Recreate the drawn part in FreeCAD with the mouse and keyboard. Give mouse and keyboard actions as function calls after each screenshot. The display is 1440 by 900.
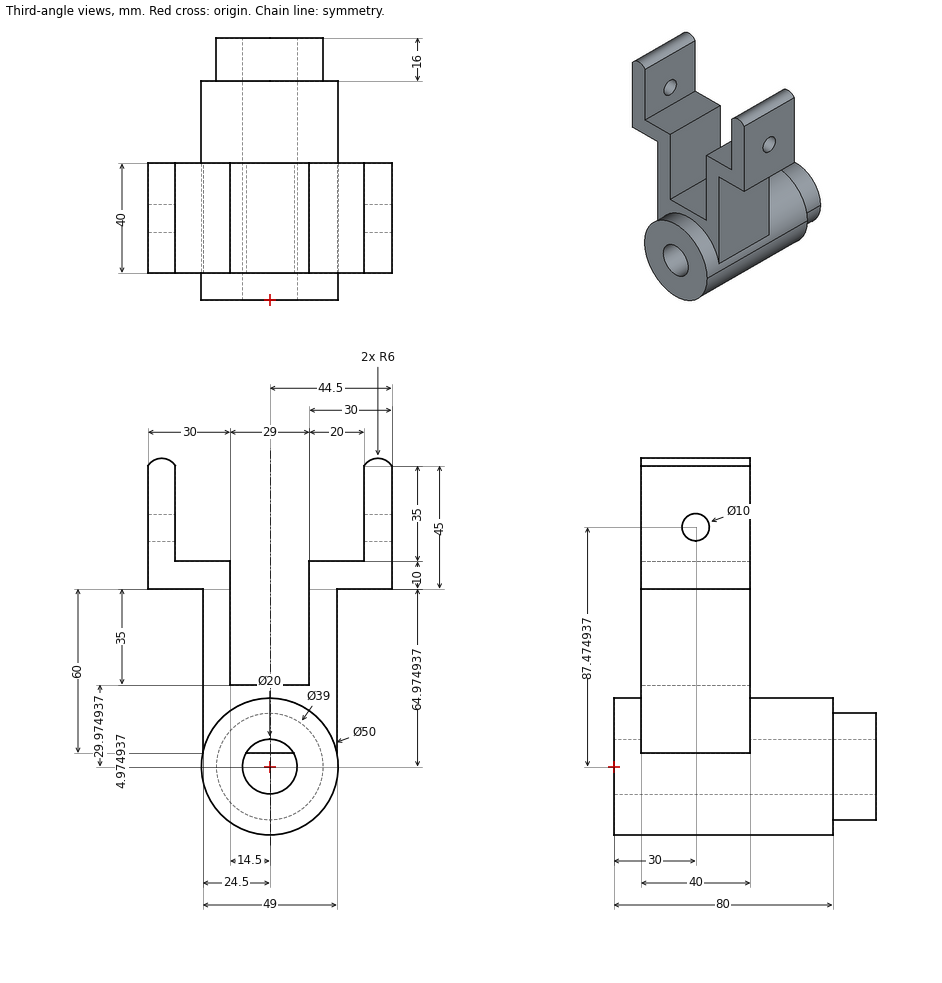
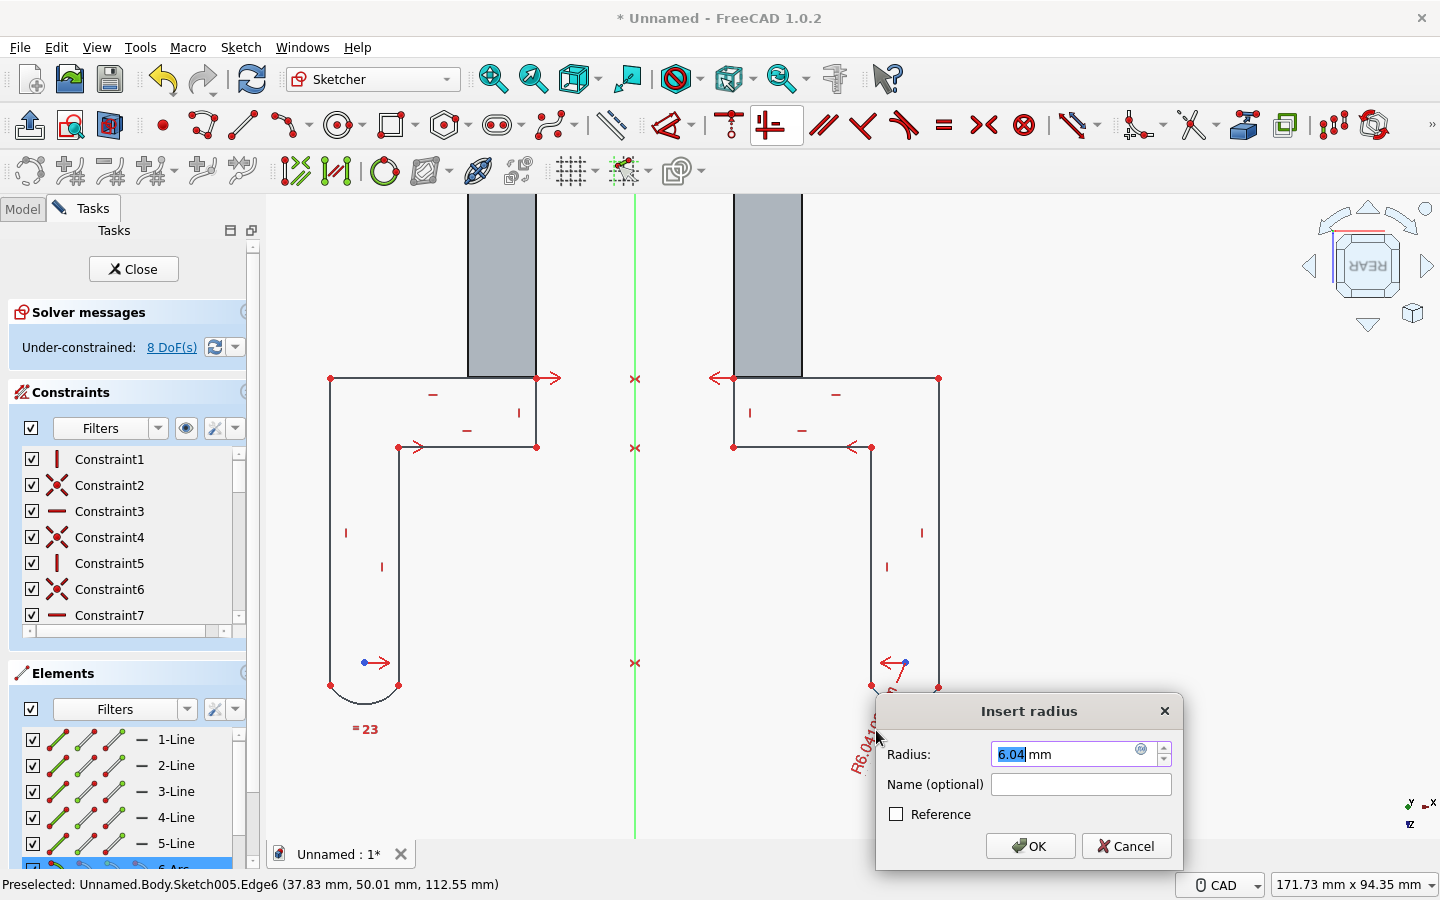
text(6)
key(Return)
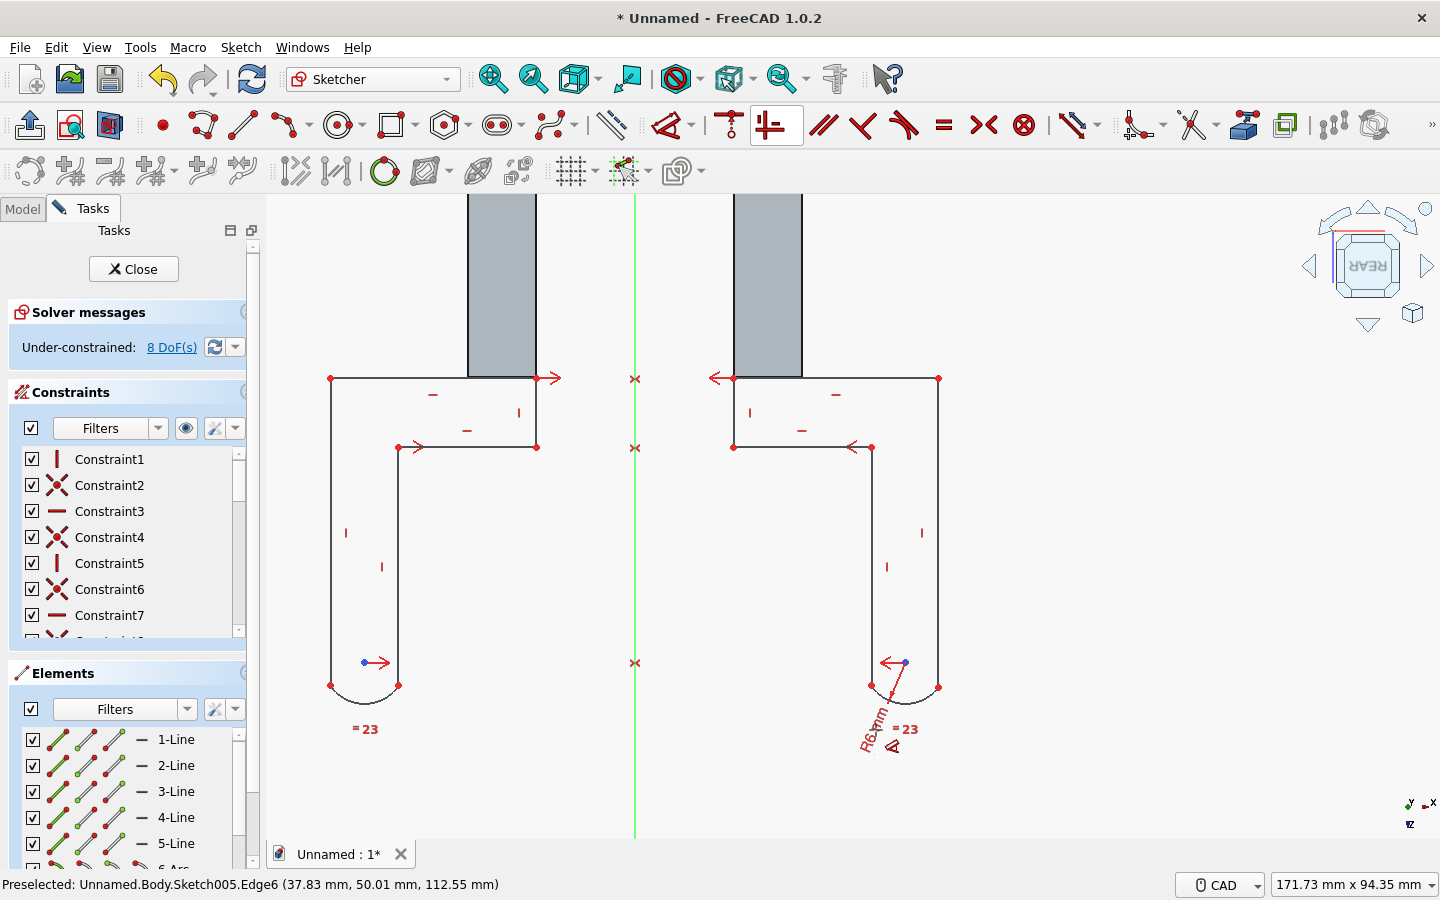
click(938, 595)
click(972, 533)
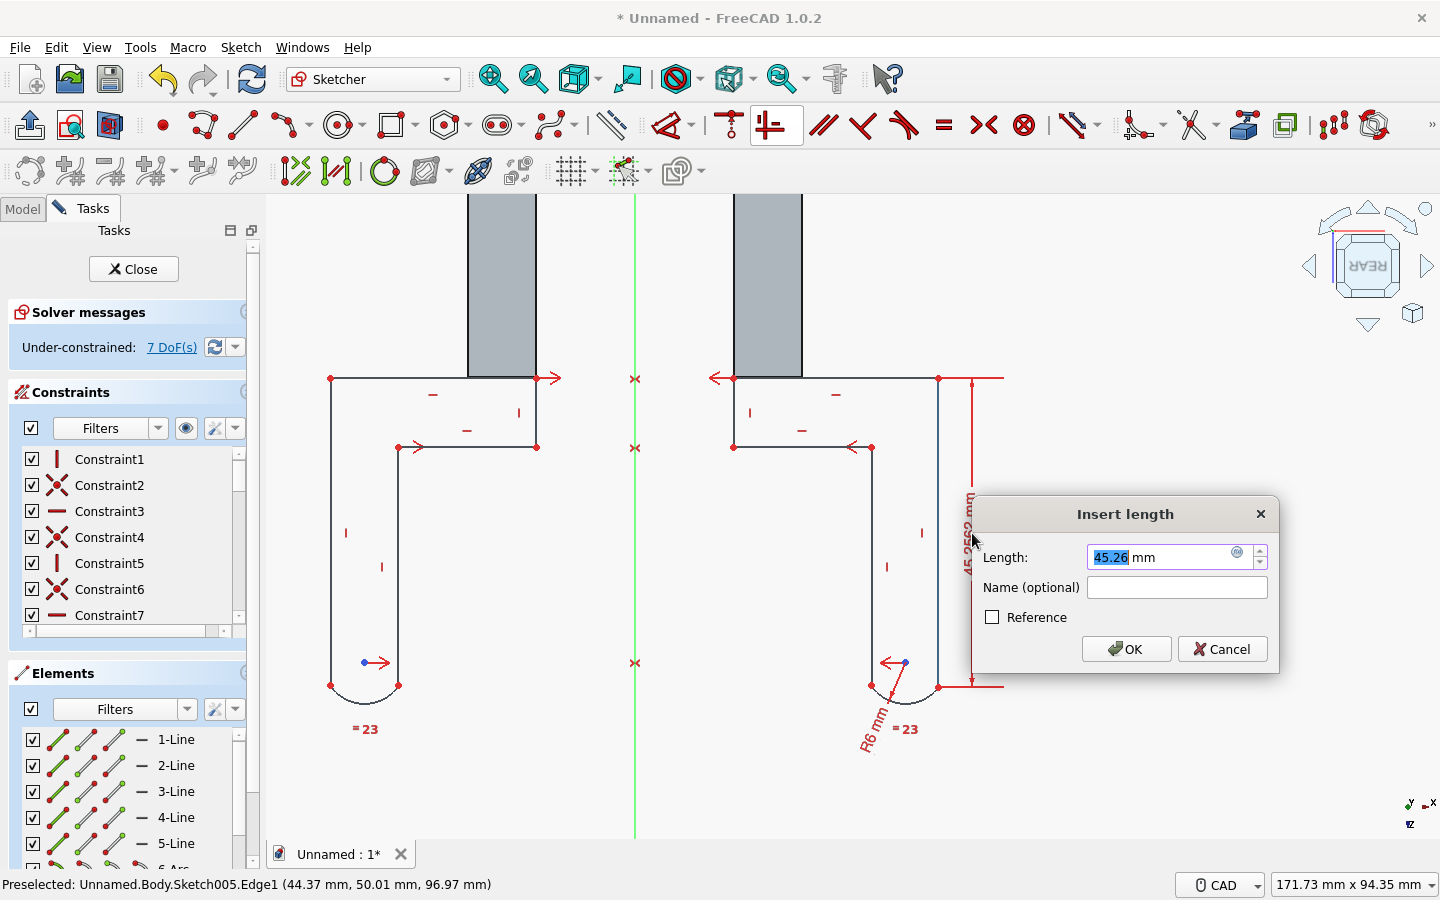
text(45)
key(Return)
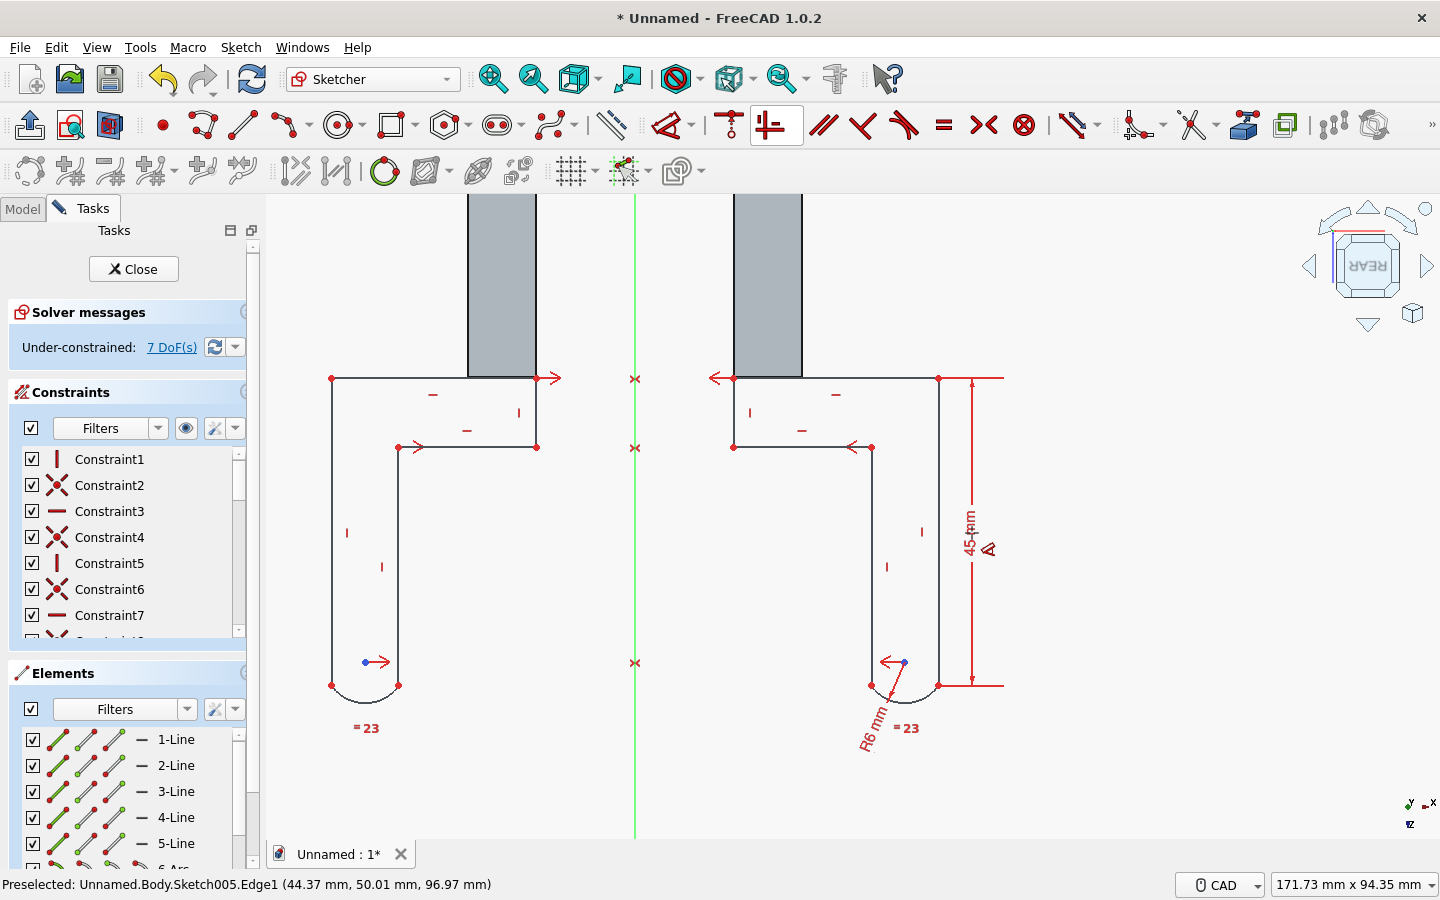
click(877, 378)
click(836, 412)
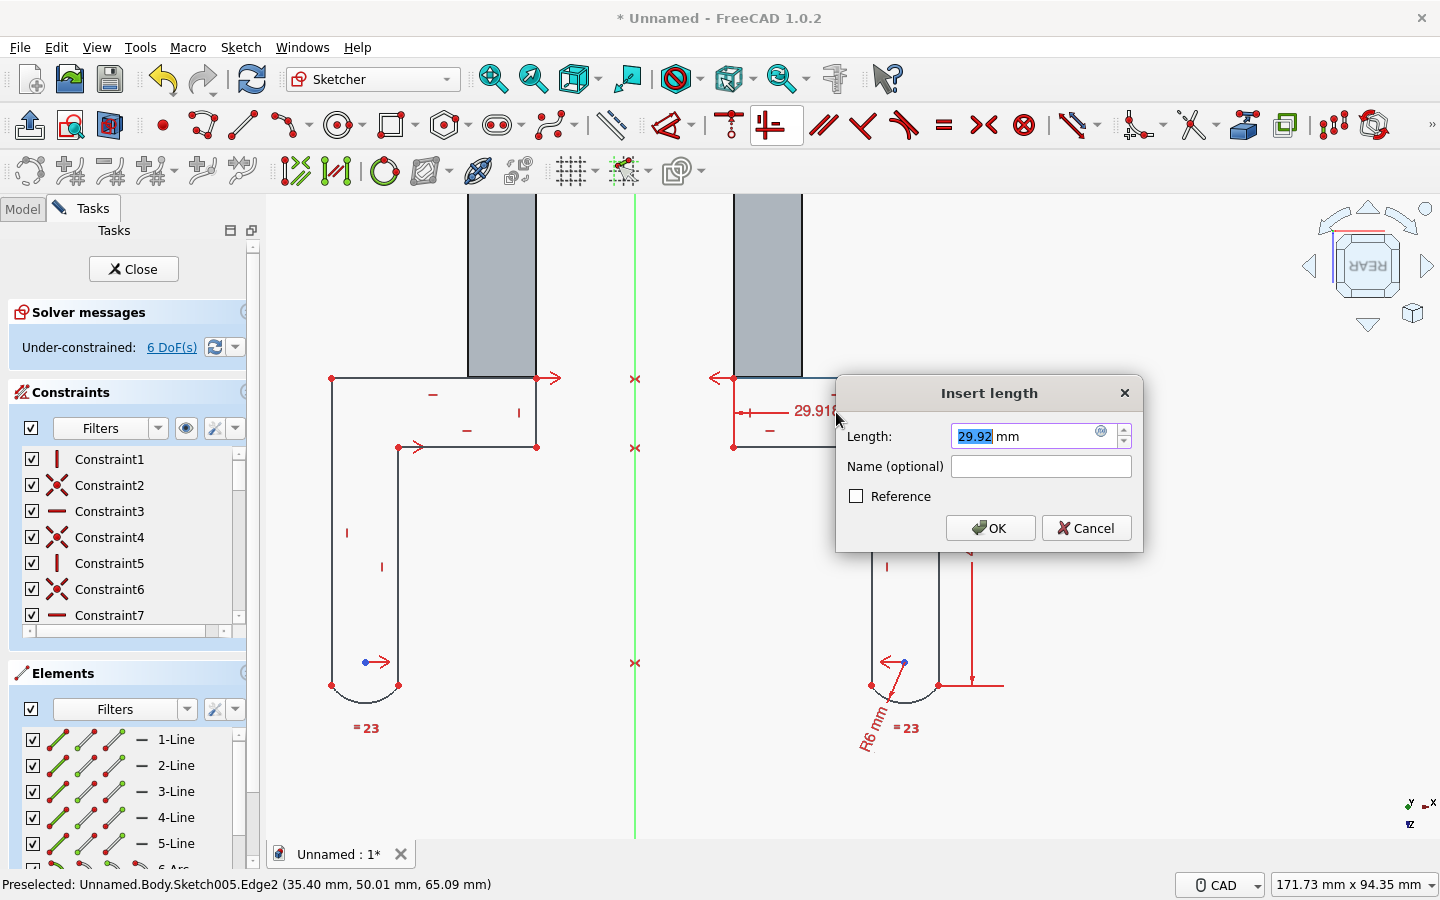
text(30)
key(Return)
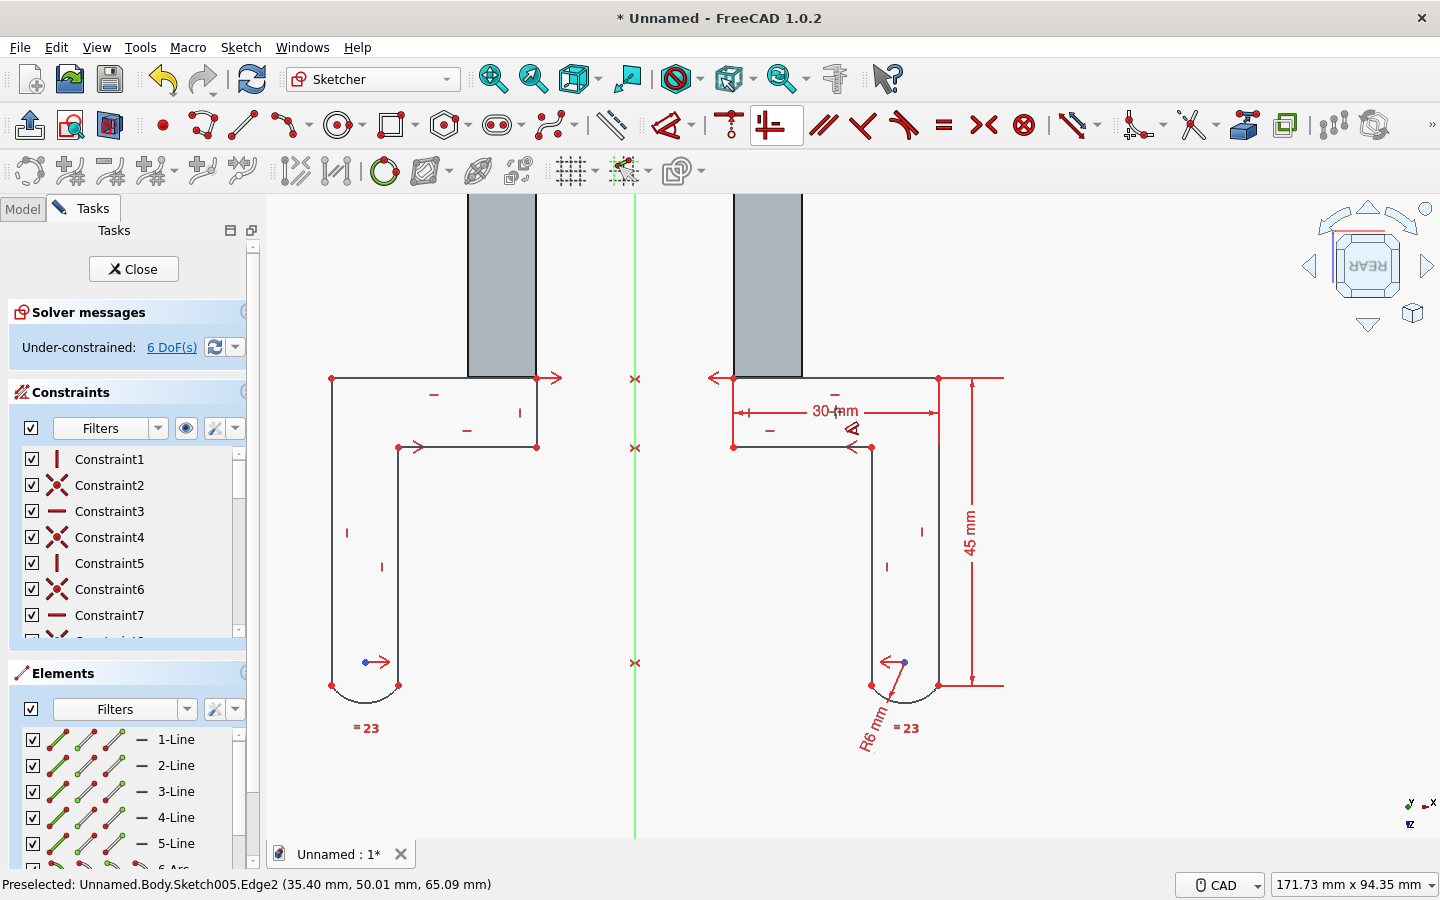
click(733, 399)
click(699, 413)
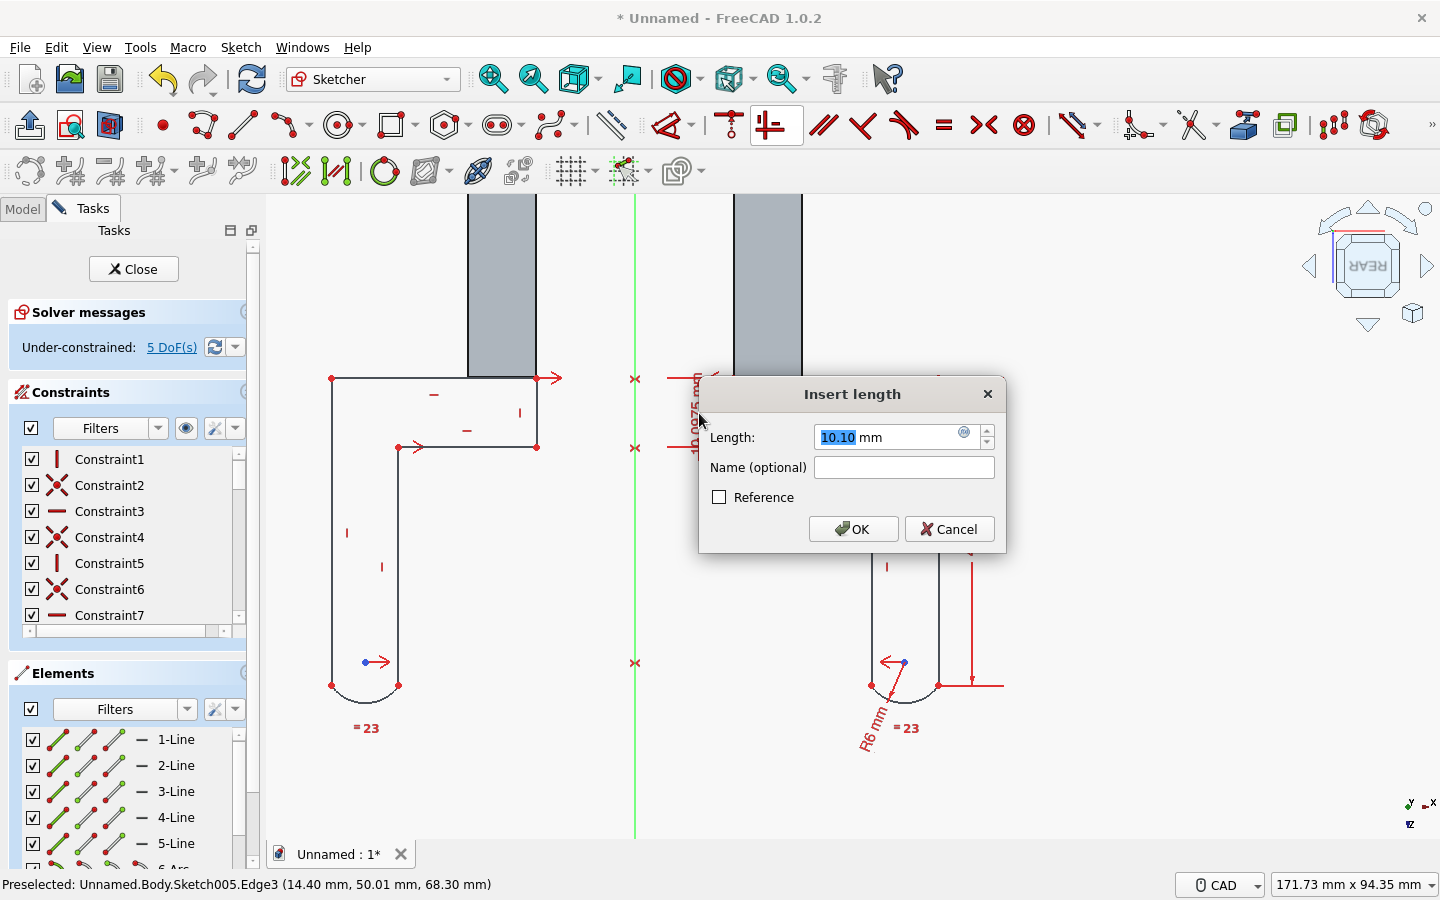
text(10)
key(Return)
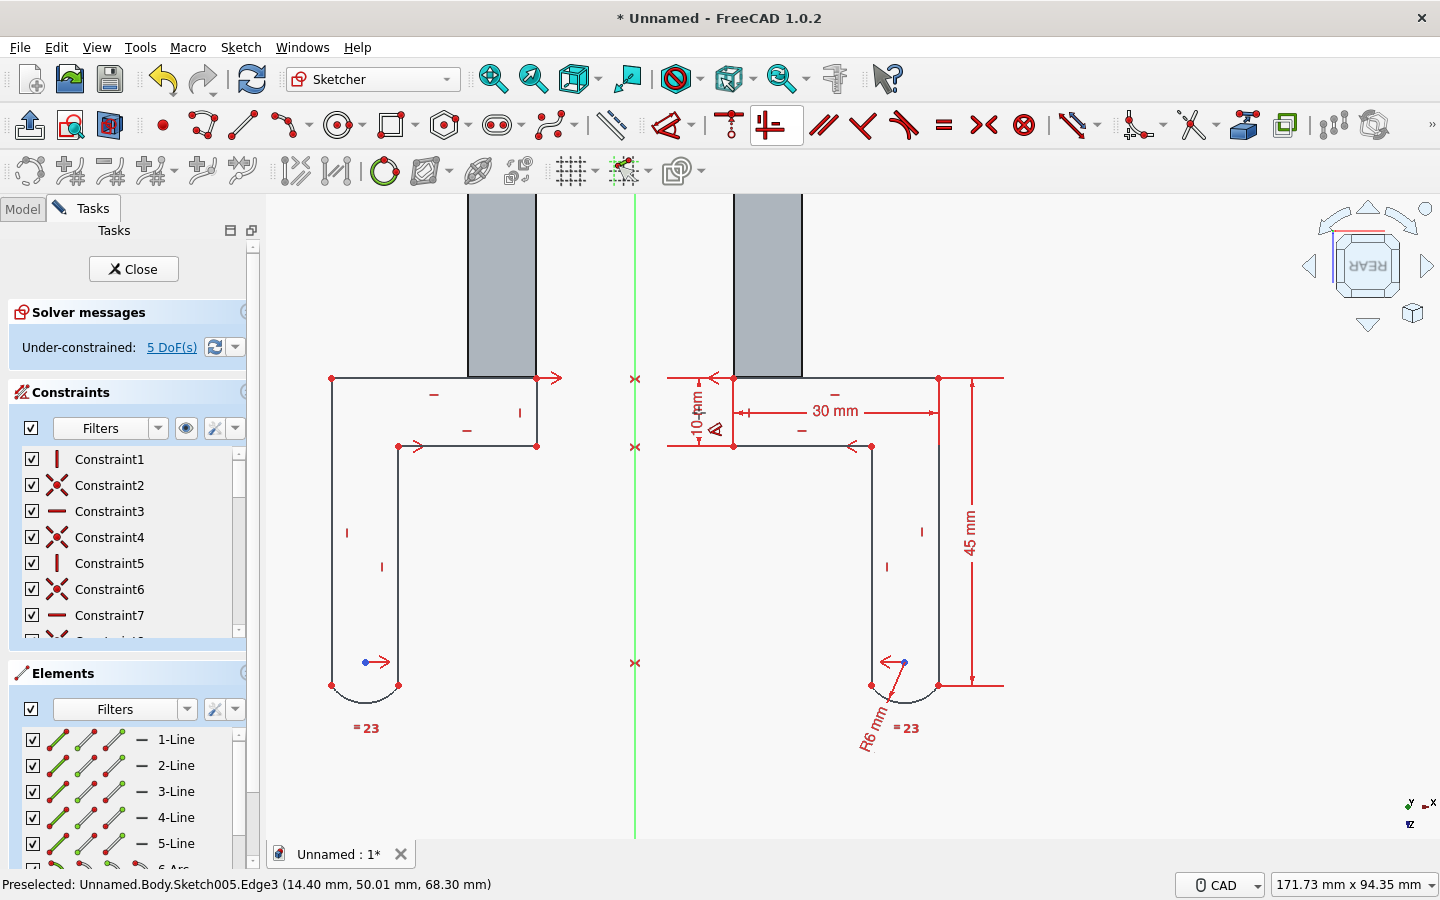
click(775, 446)
click(802, 480)